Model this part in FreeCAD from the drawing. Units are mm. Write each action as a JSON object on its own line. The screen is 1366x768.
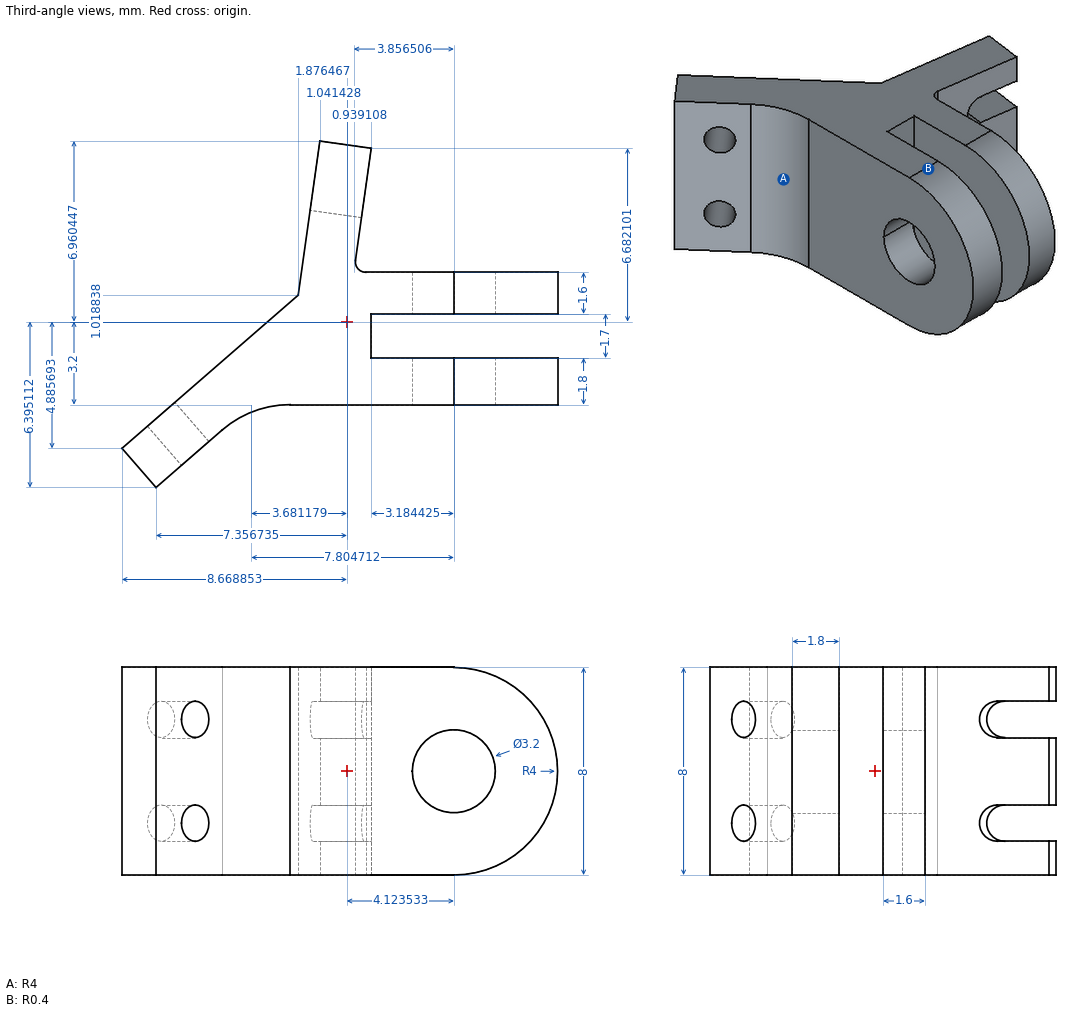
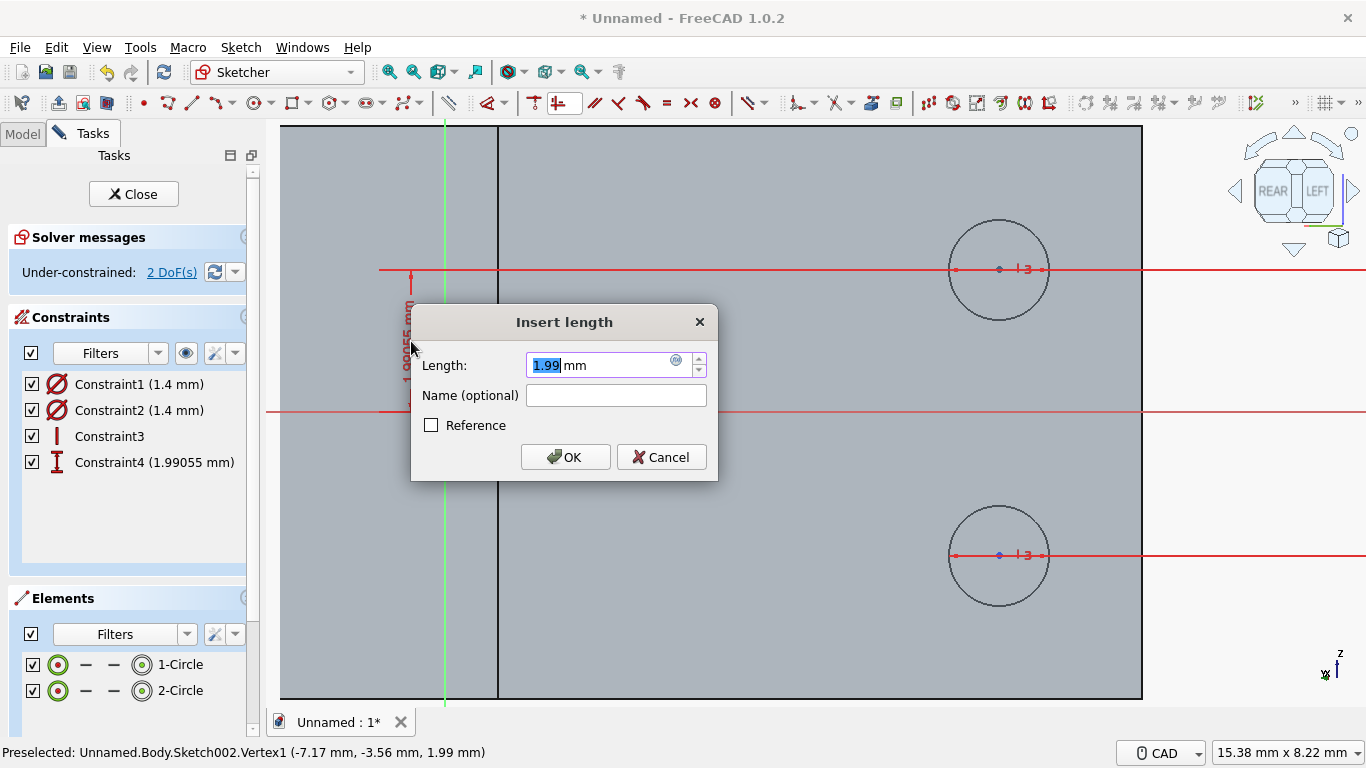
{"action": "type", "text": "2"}
{"action": "key", "text": "Return"}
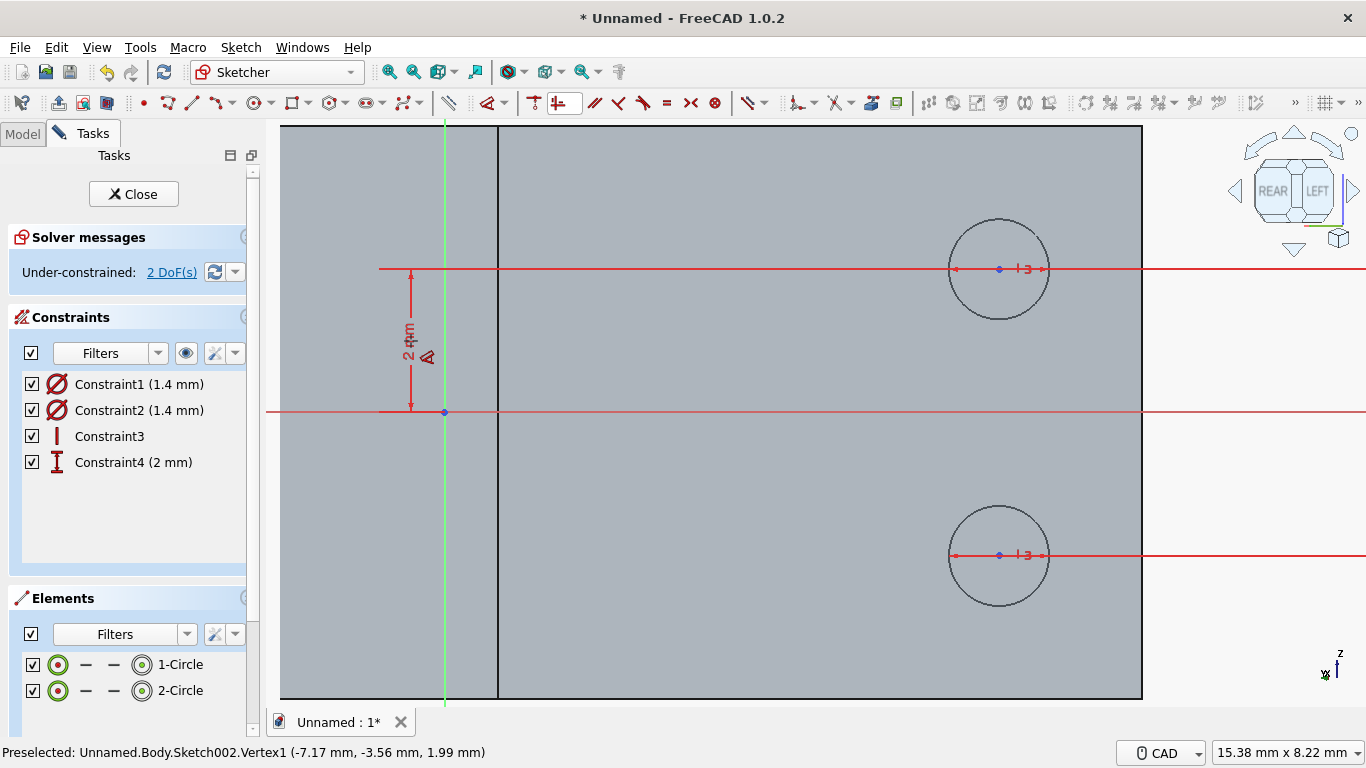
{"action": "left_click", "coordinate": [999, 556]}
{"action": "left_click", "coordinate": [411, 484]}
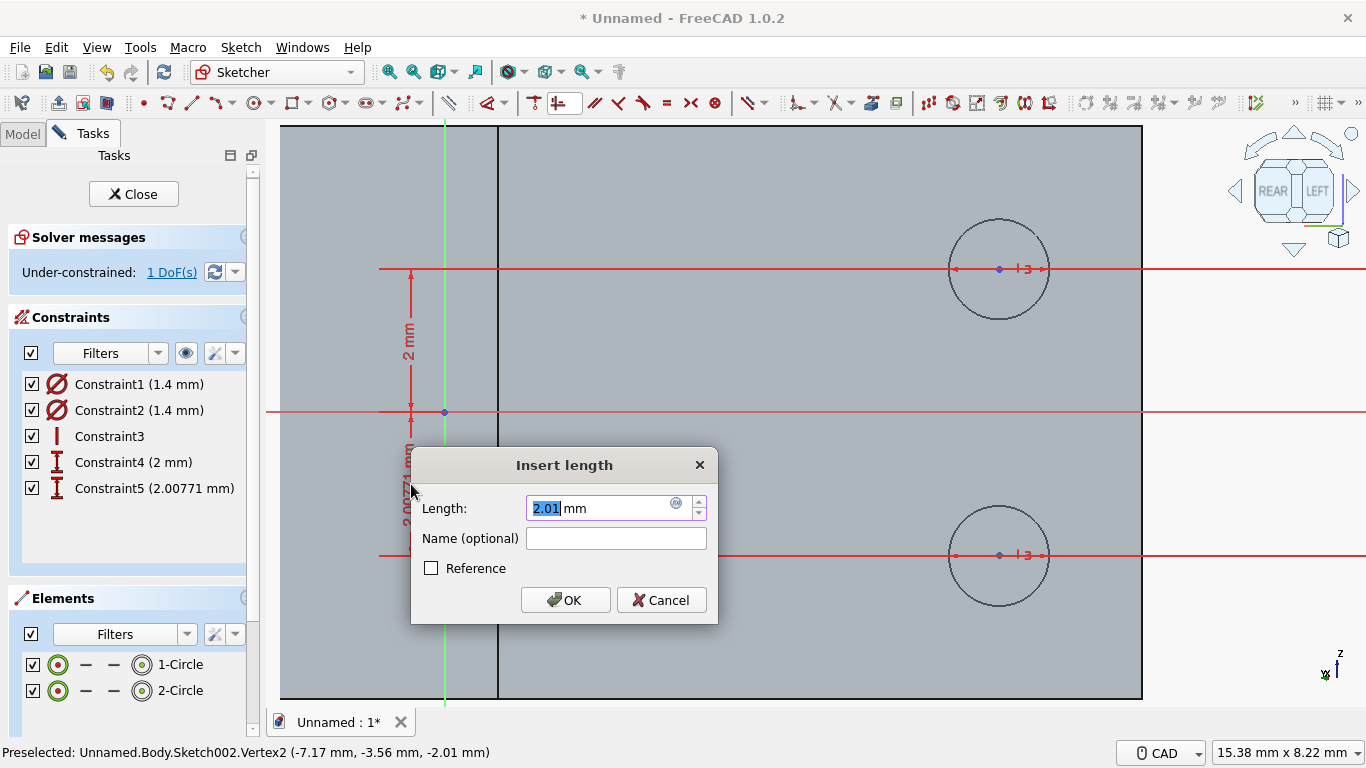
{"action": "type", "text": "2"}
{"action": "key", "text": "Return"}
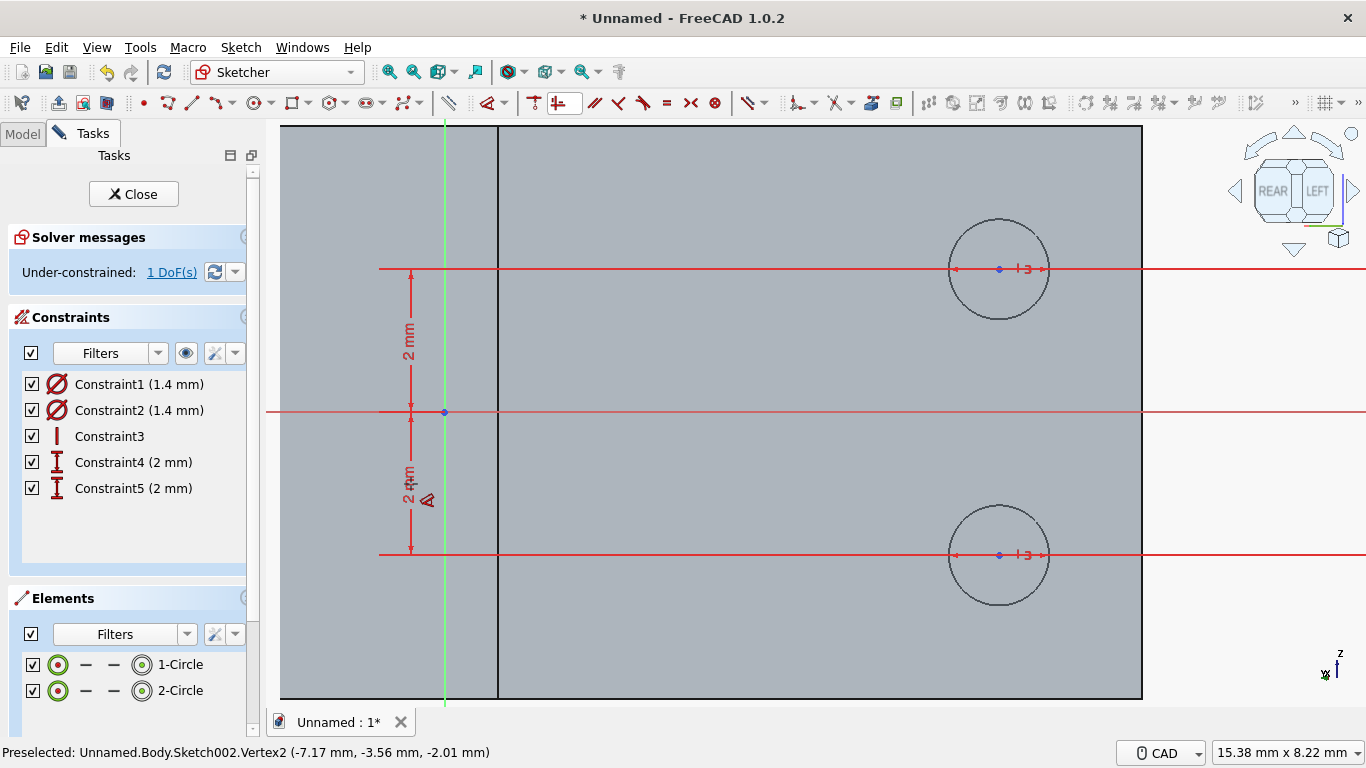
{"action": "left_click", "coordinate": [999, 269]}
{"action": "left_click", "coordinate": [722, 235]}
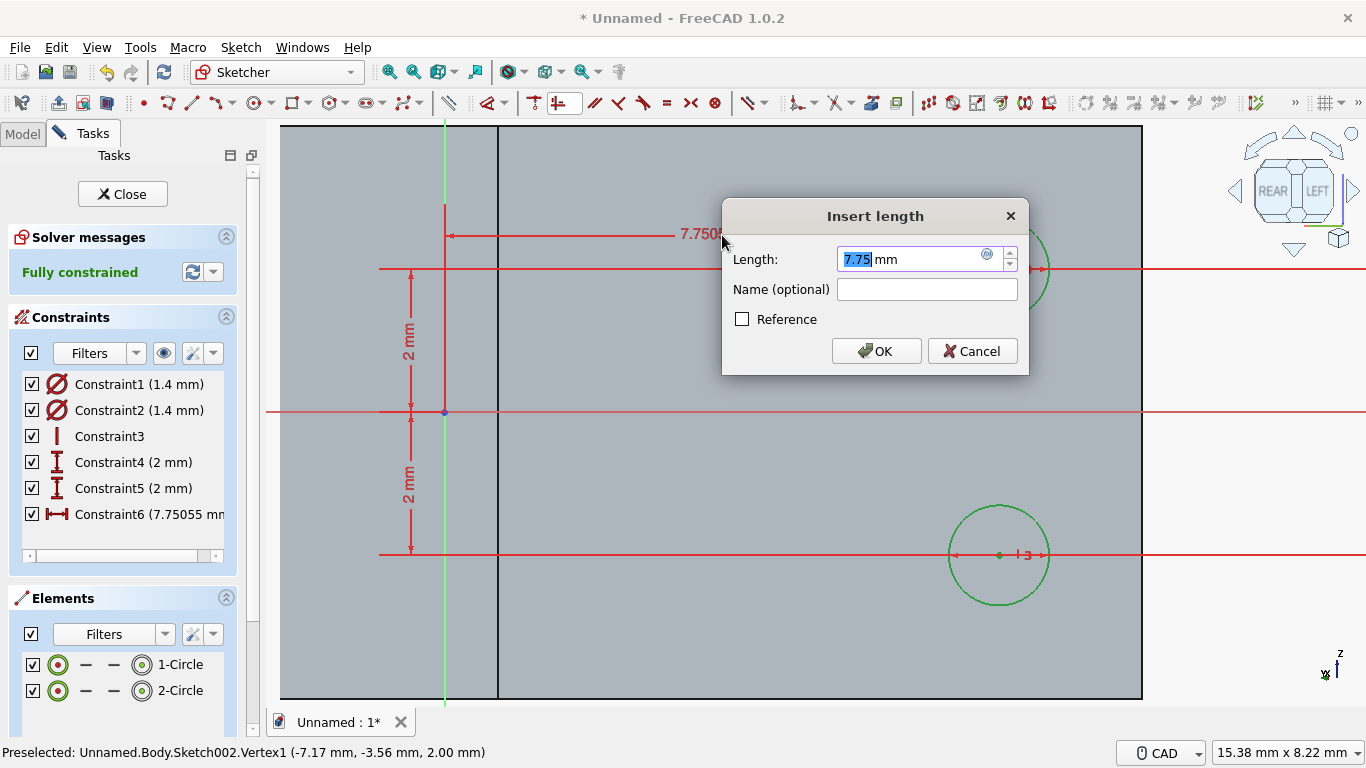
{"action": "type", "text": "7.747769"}
{"action": "key", "text": "Return"}
{"action": "key", "text": "Escape"}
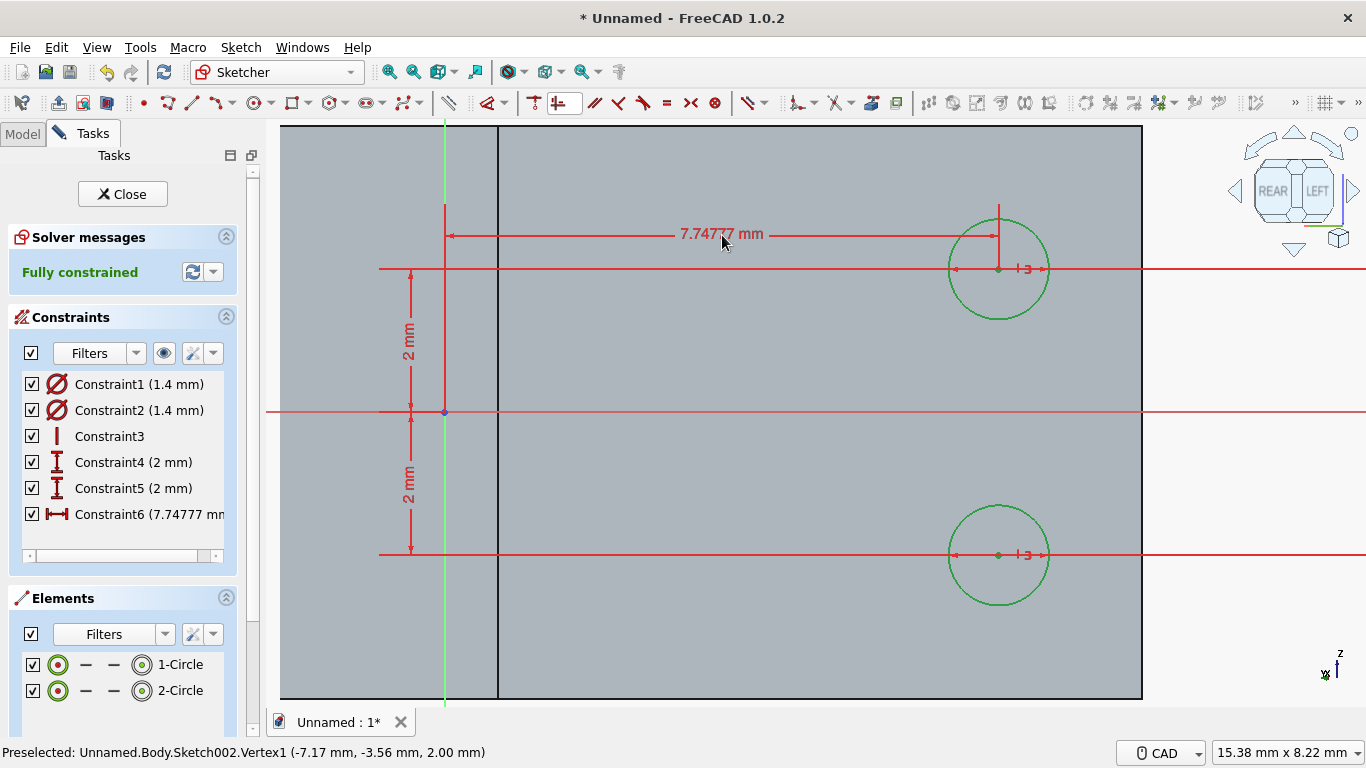
{"action": "left_click", "coordinate": [123, 194]}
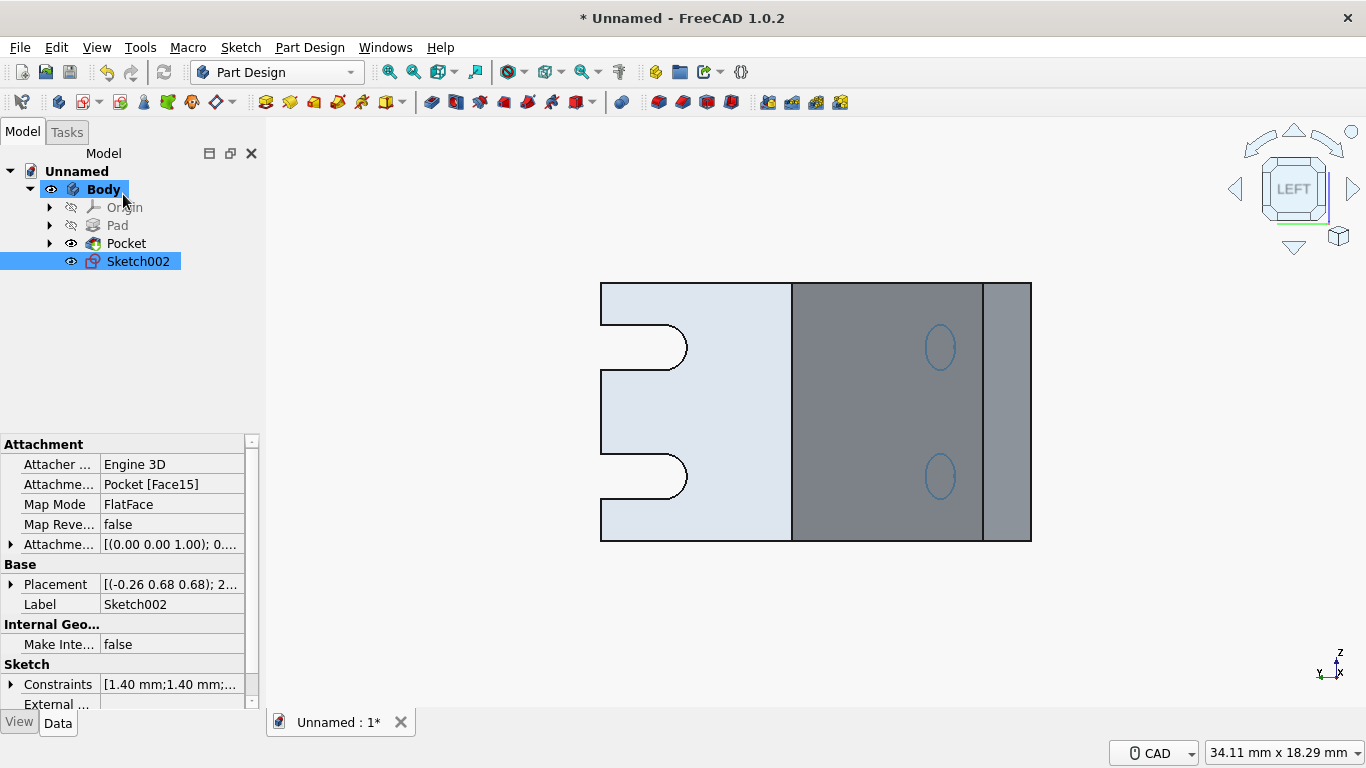
{"action": "left_click", "coordinate": [432, 102]}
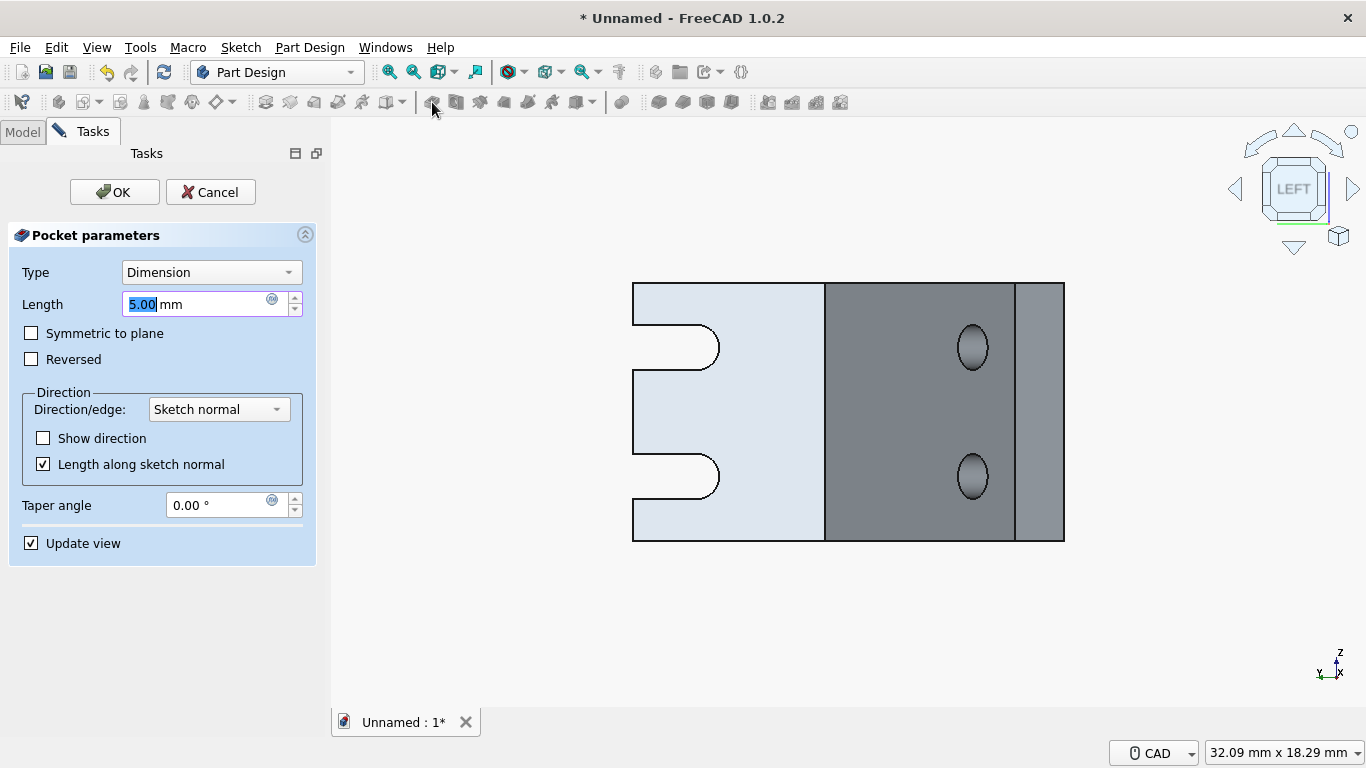
{"action": "left_click", "coordinate": [212, 272]}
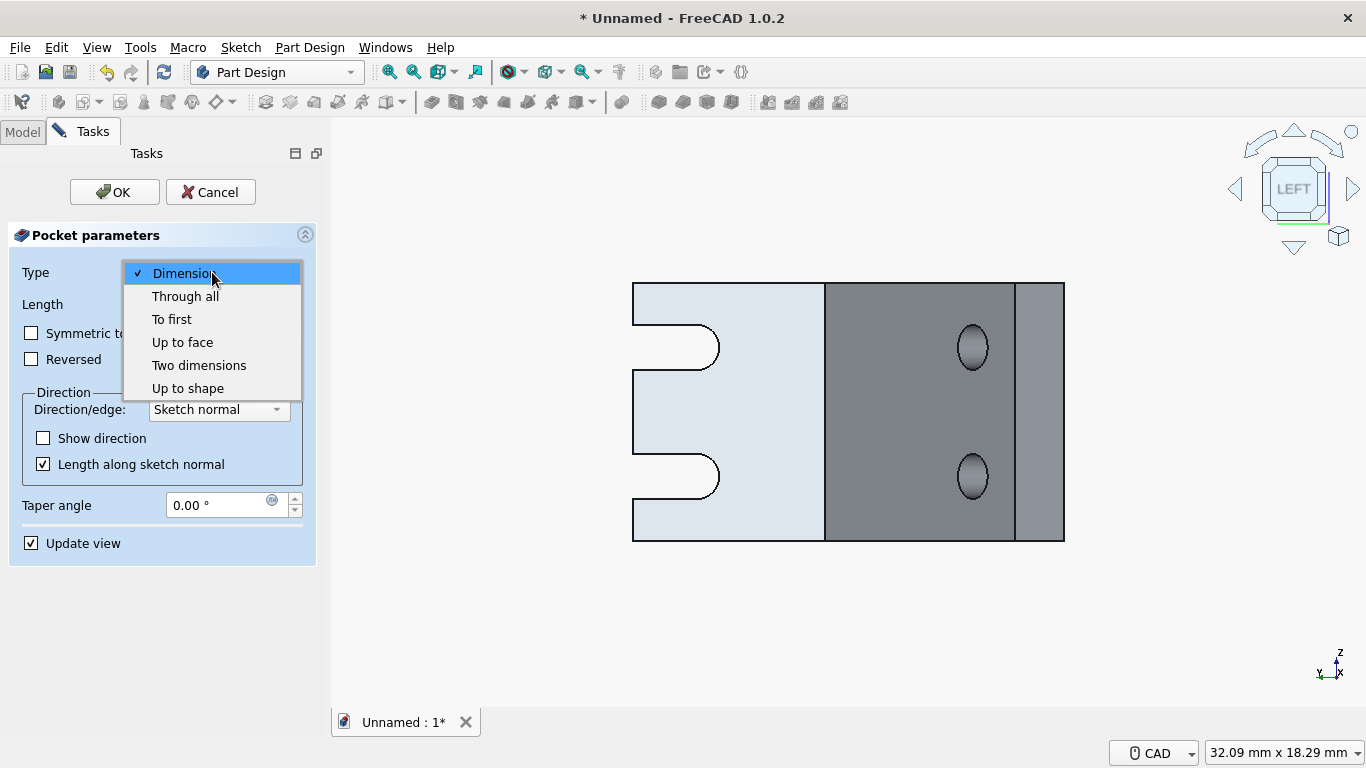
{"action": "left_click", "coordinate": [212, 296]}